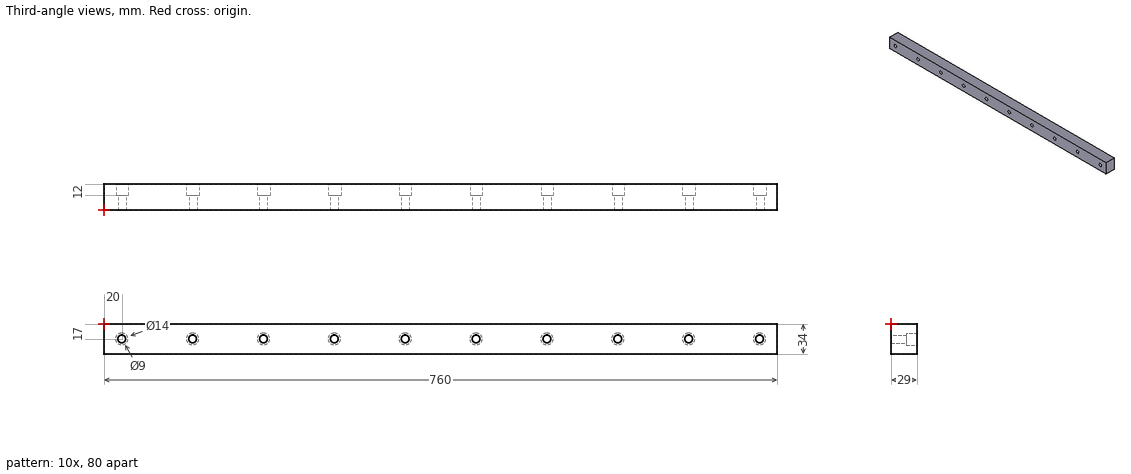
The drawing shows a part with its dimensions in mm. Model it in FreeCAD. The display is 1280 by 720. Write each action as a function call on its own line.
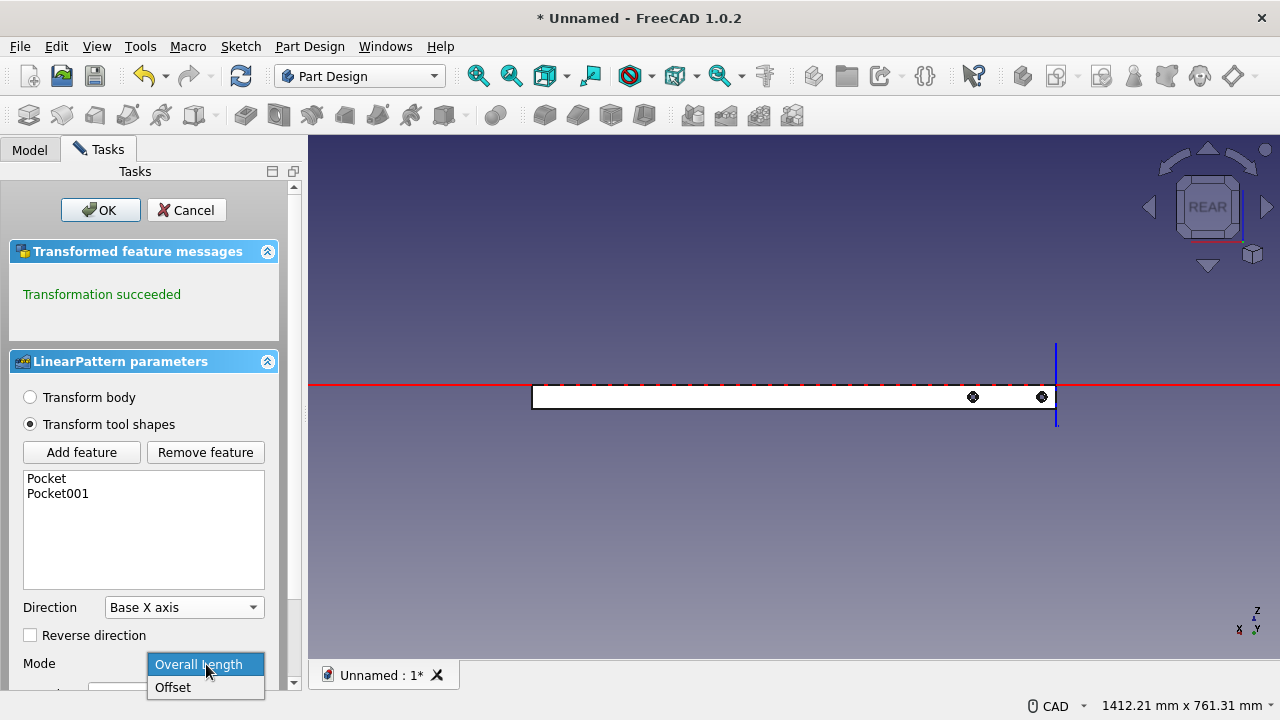
click(204, 688)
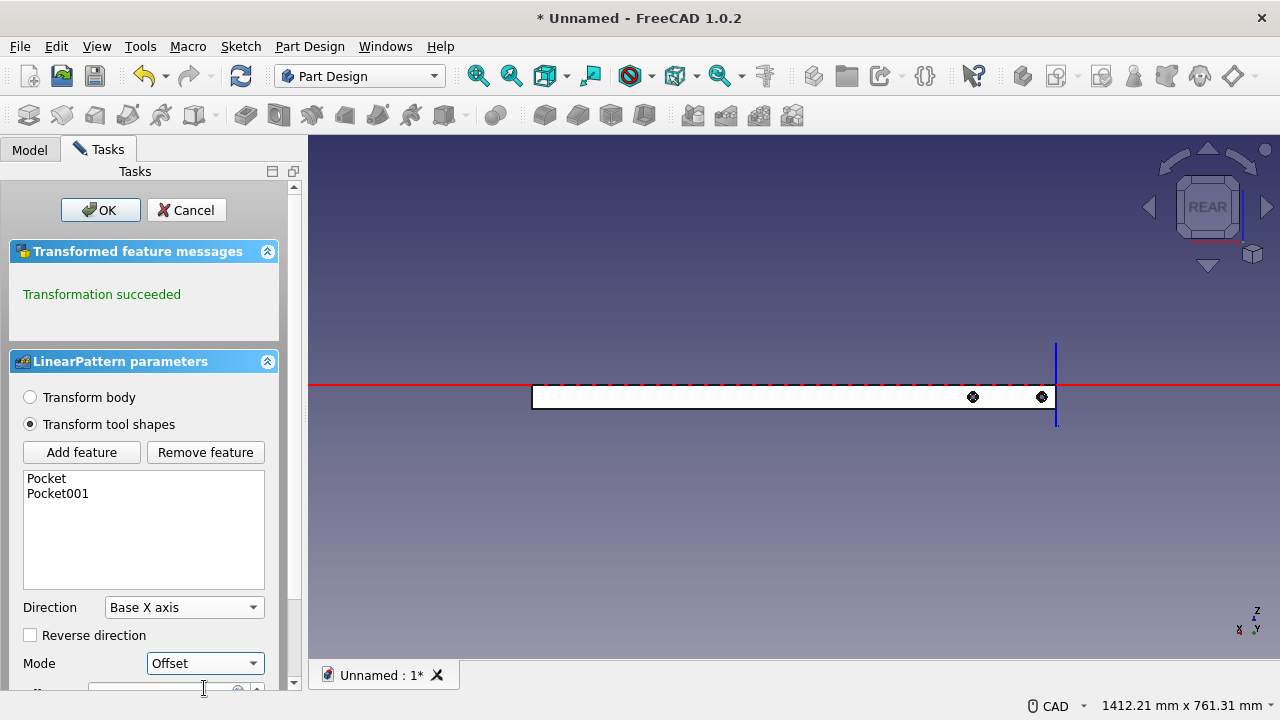
scroll(294, 436, down, 2)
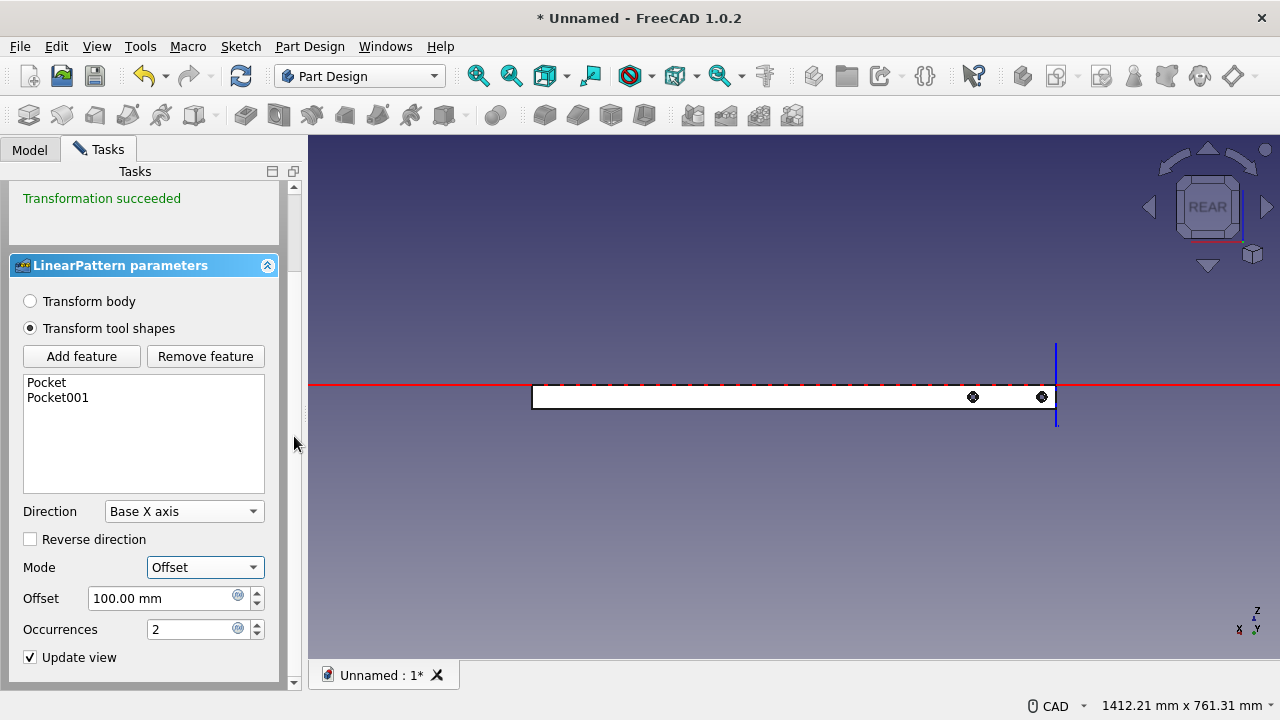
triple_click(170, 598)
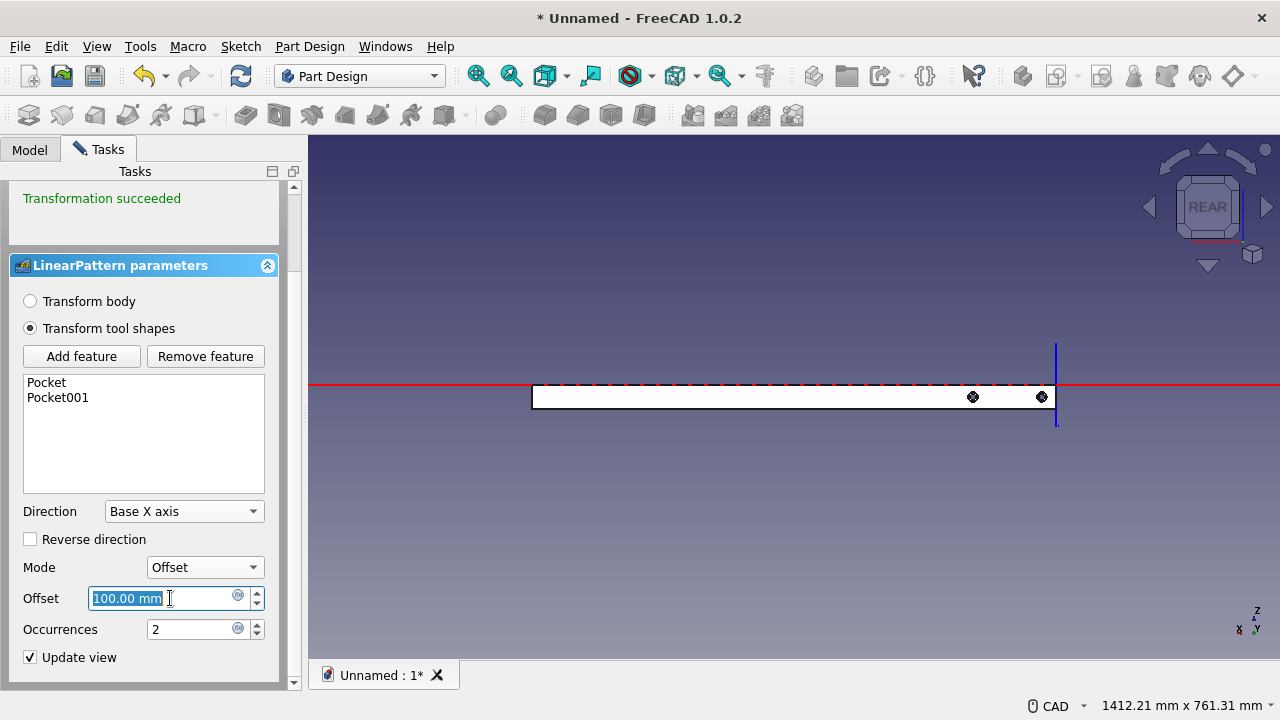
text(80)
key(Tab)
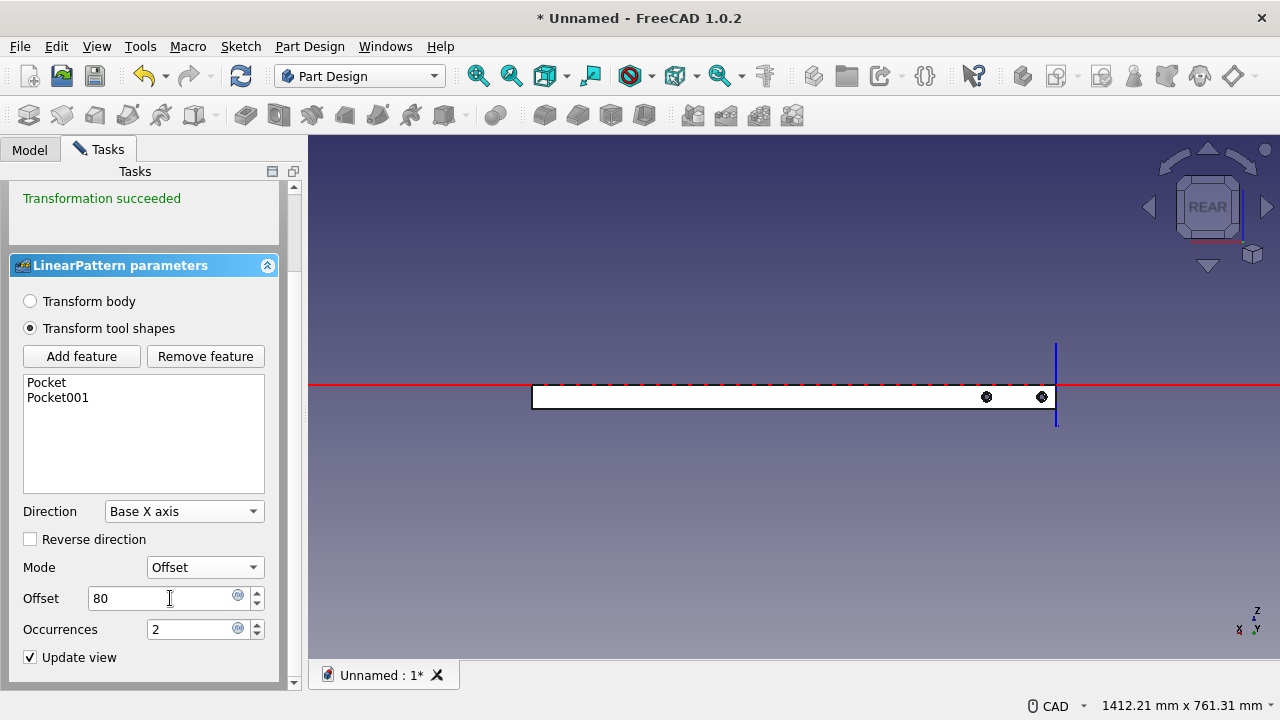
triple_click(199, 630)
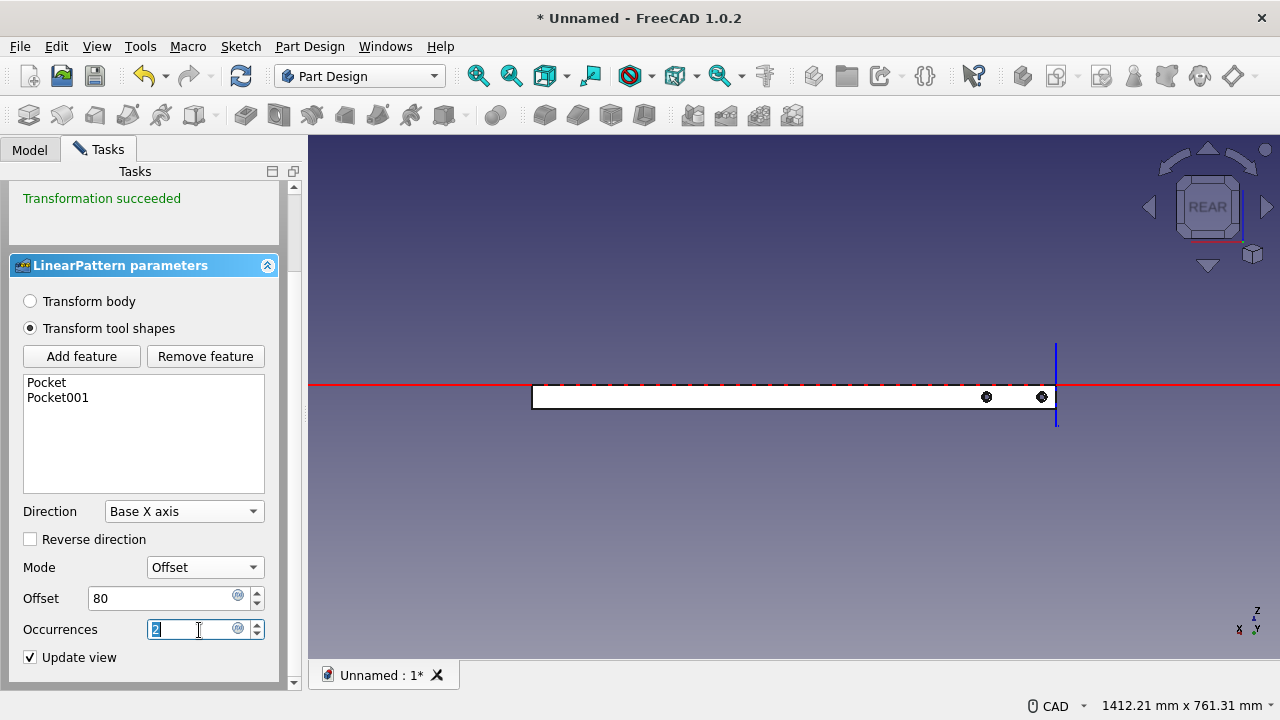
text(10)
key(Tab)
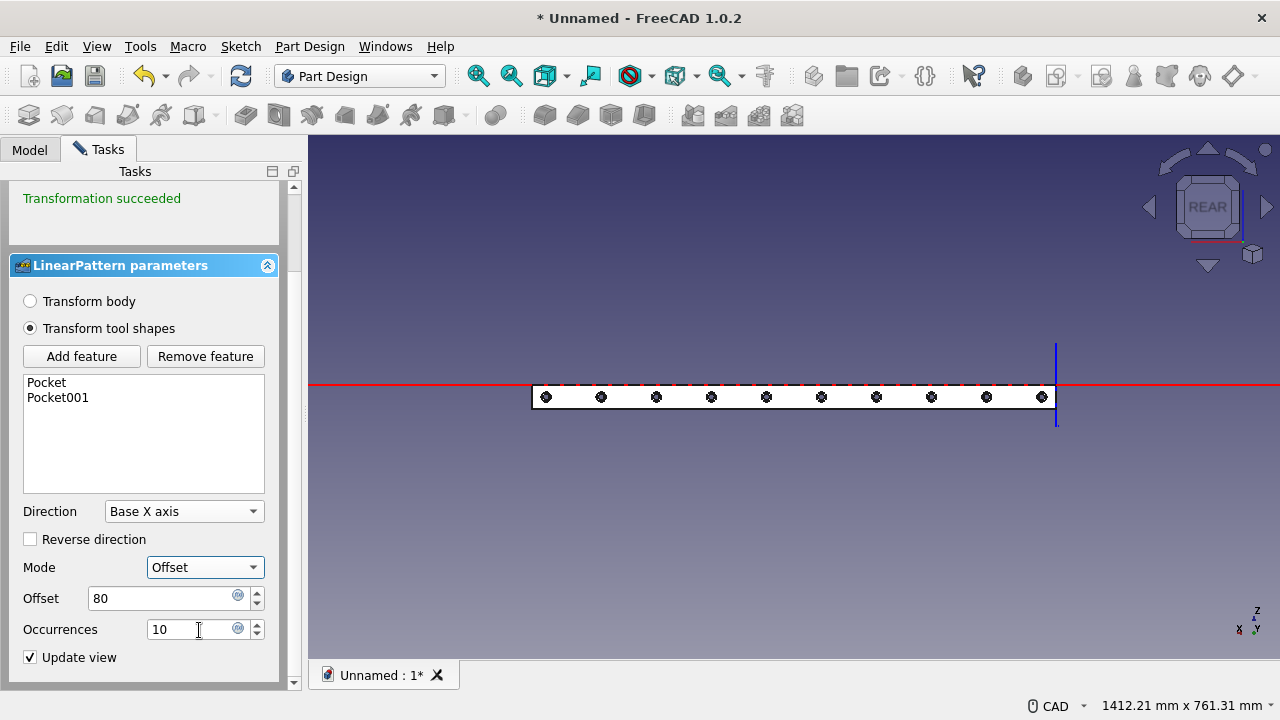
scroll(294, 436, up, 3)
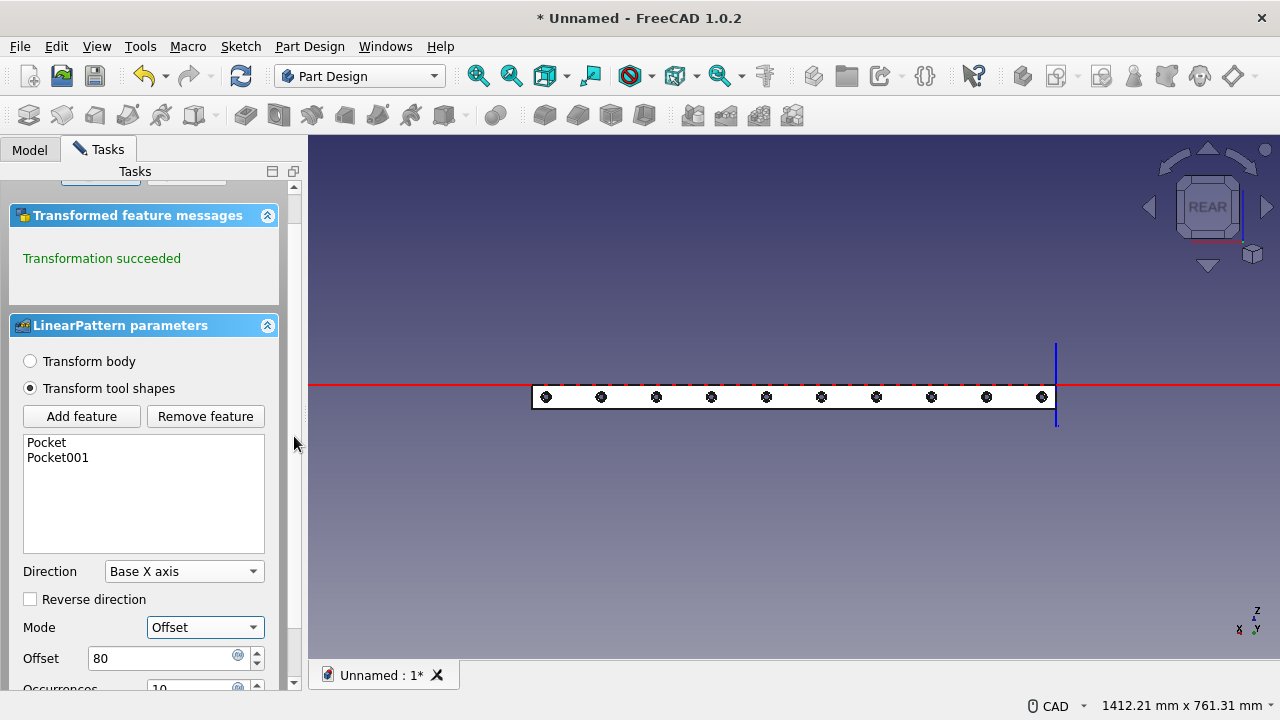
click(101, 210)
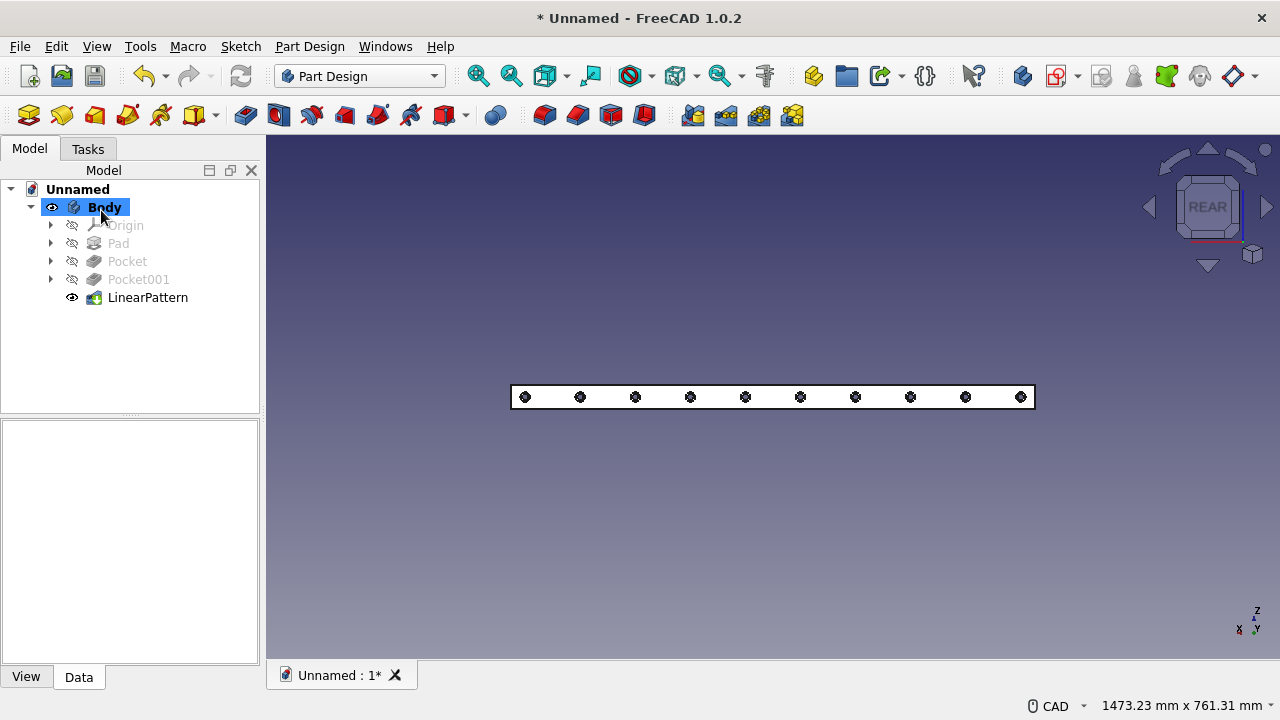
key(0)